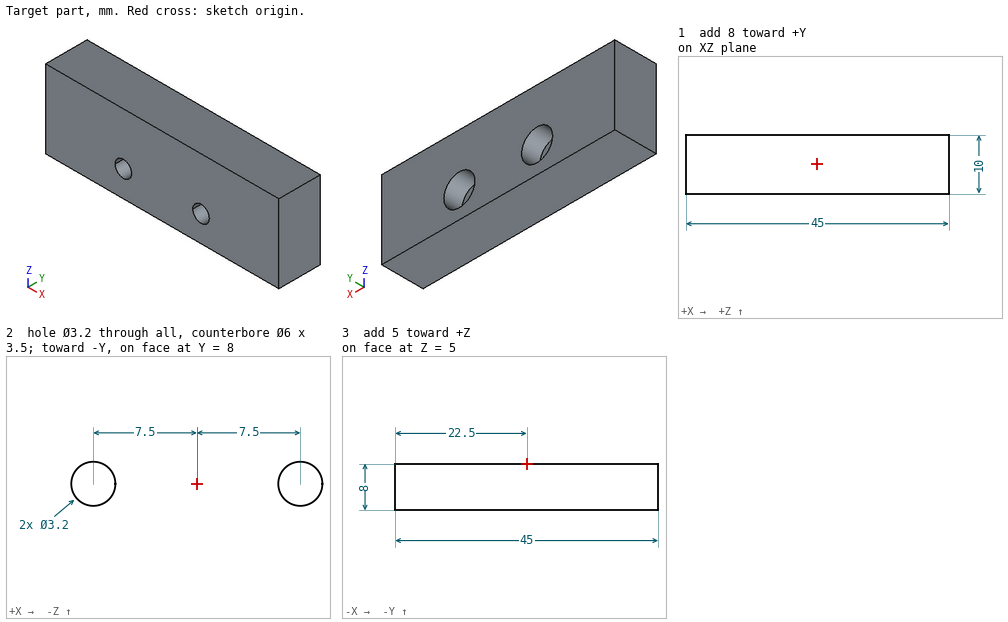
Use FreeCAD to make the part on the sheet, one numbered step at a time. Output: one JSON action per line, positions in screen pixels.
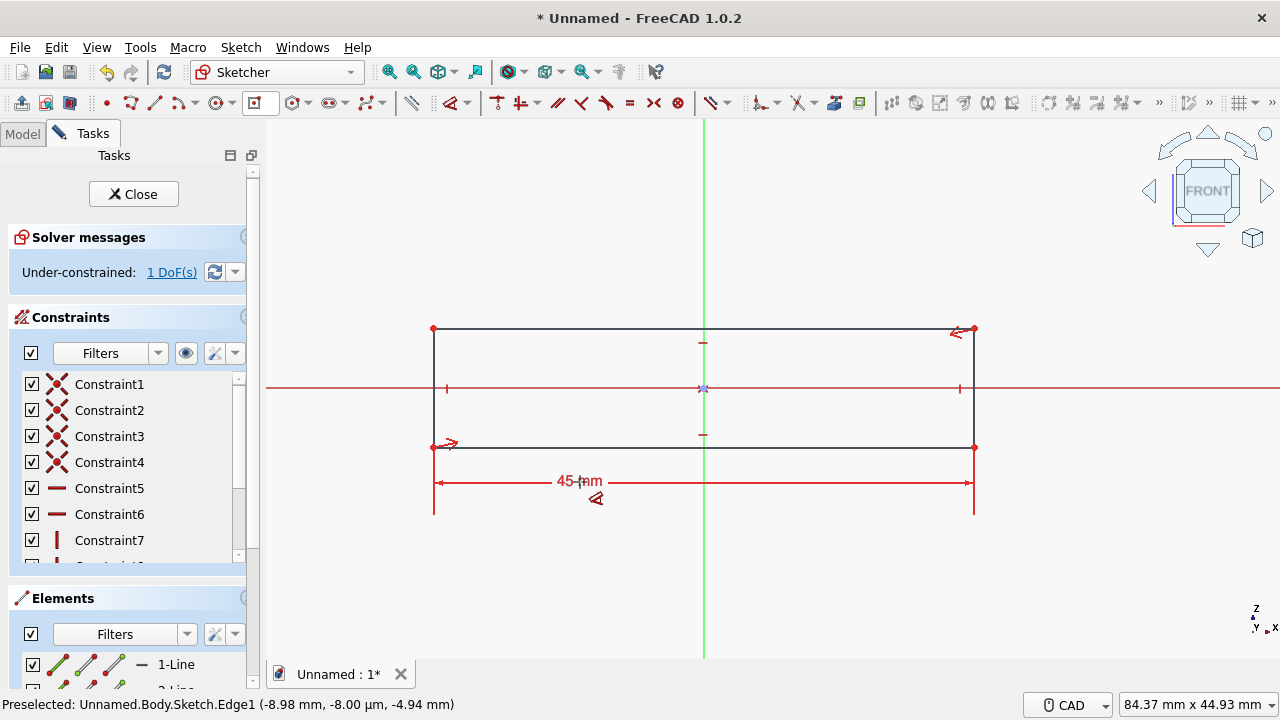
{"action": "left_click", "coordinate": [974, 412]}
{"action": "left_click", "coordinate": [1008, 361]}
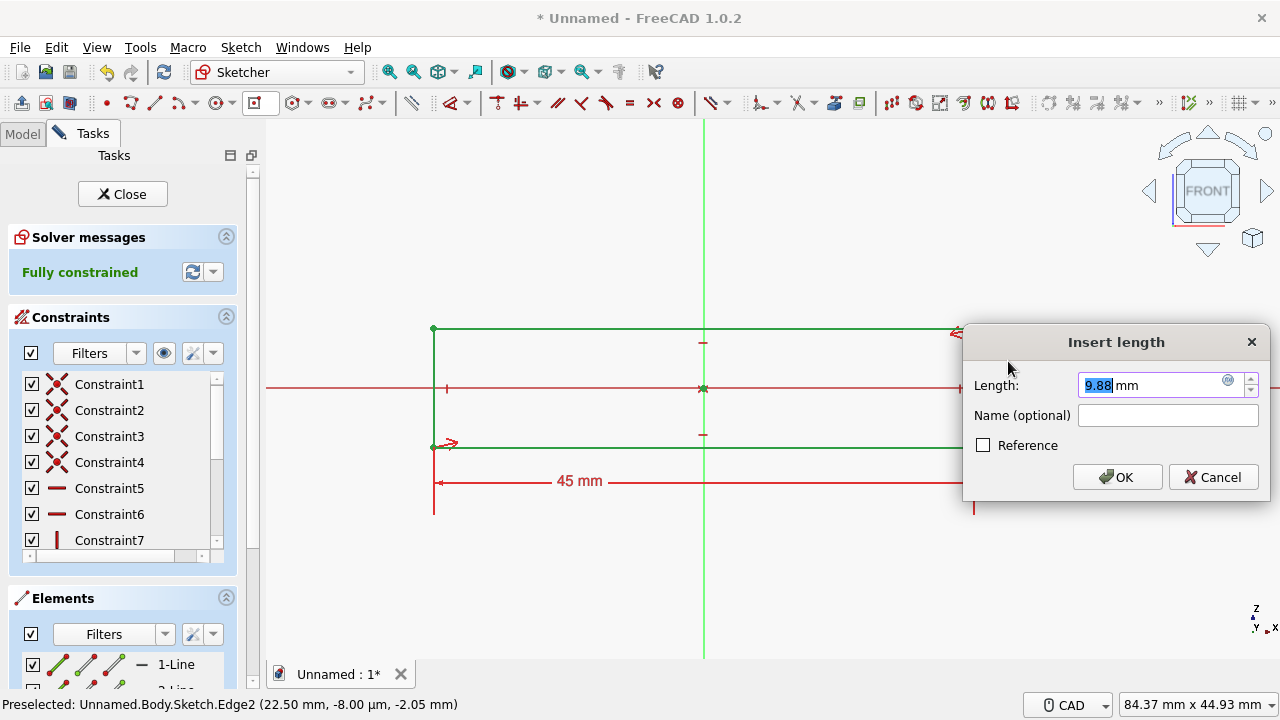
{"action": "type", "text": "10"}
{"action": "key", "text": "Return"}
{"action": "key", "text": "Escape"}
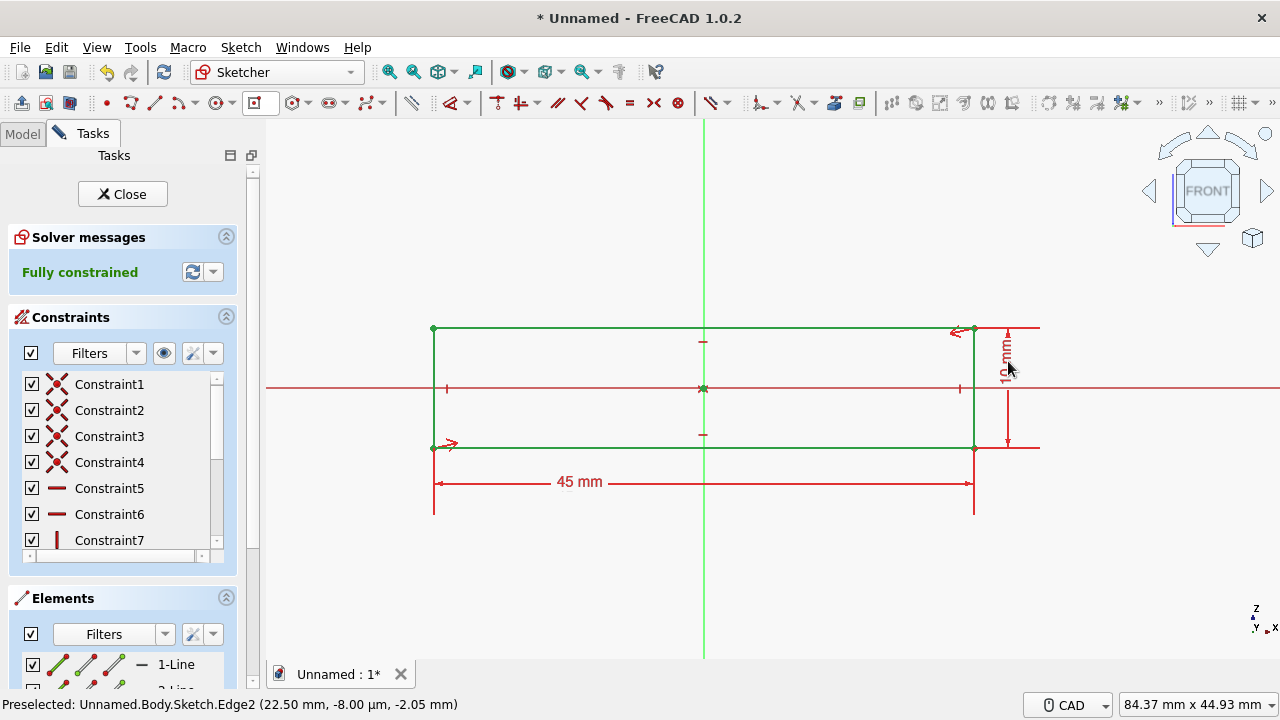
{"action": "left_click", "coordinate": [123, 194]}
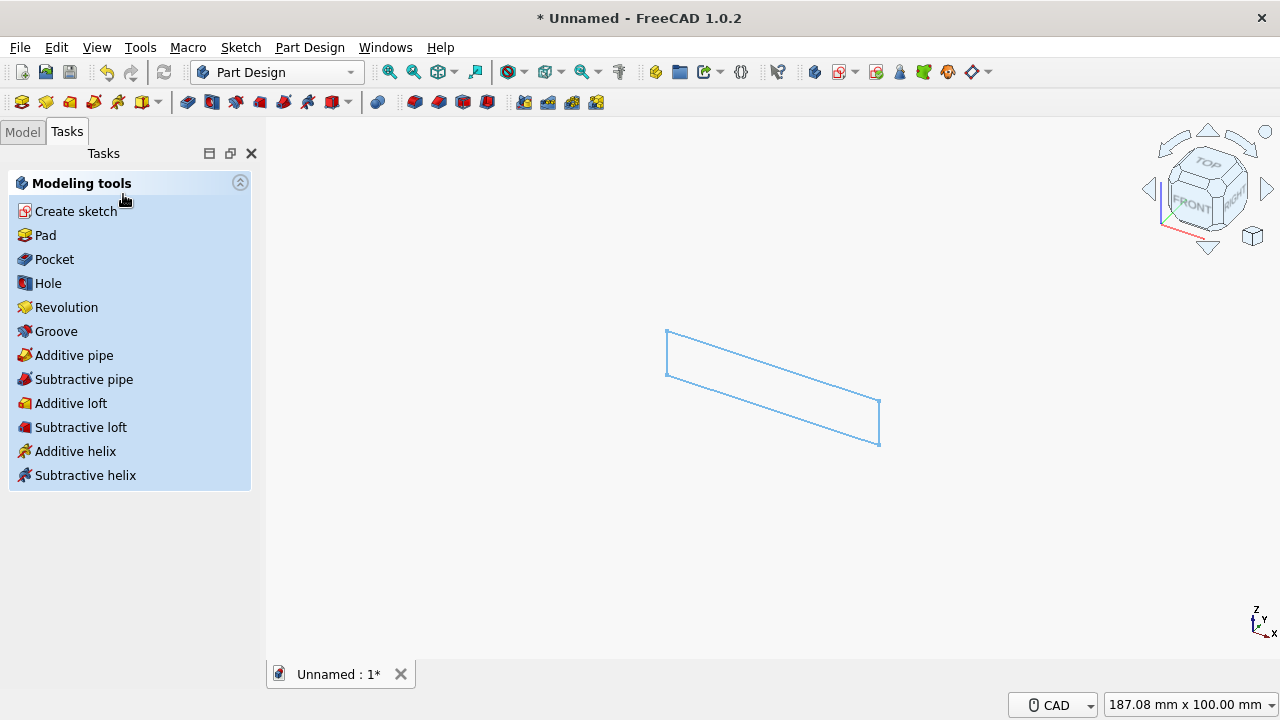
{"action": "left_click", "coordinate": [22, 102]}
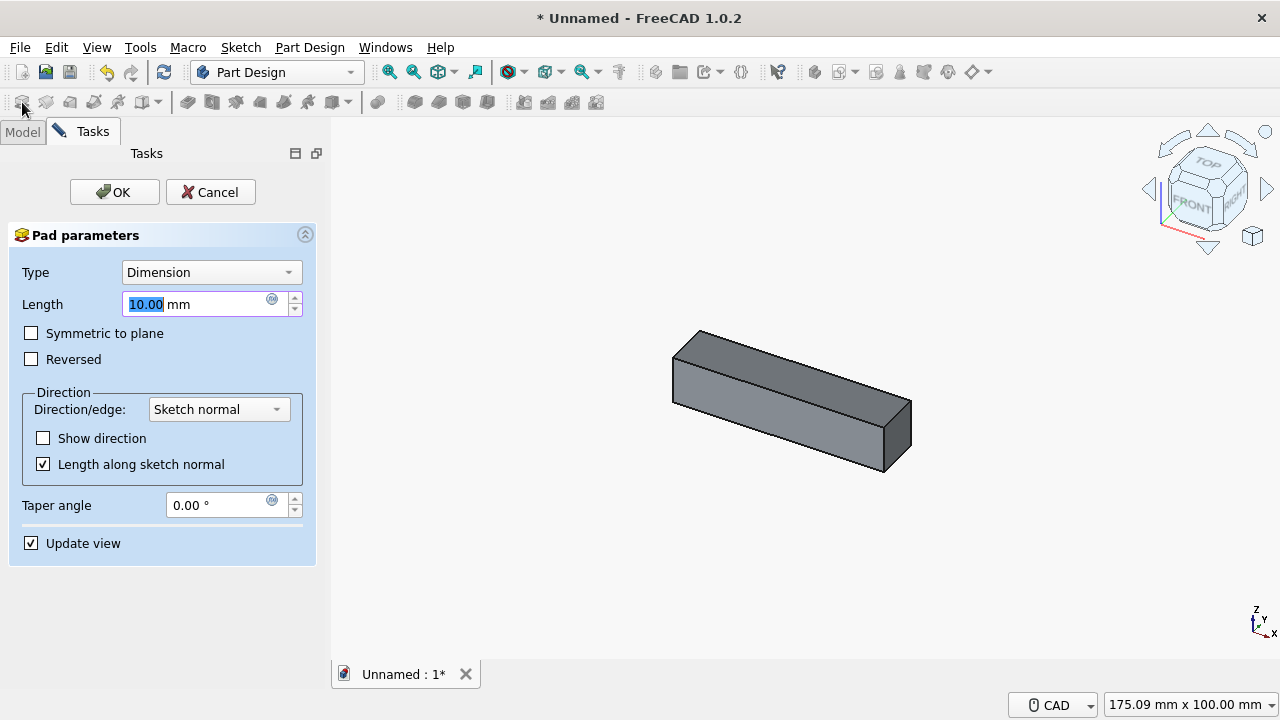
{"action": "type", "text": "8"}
{"action": "key", "text": "Tab"}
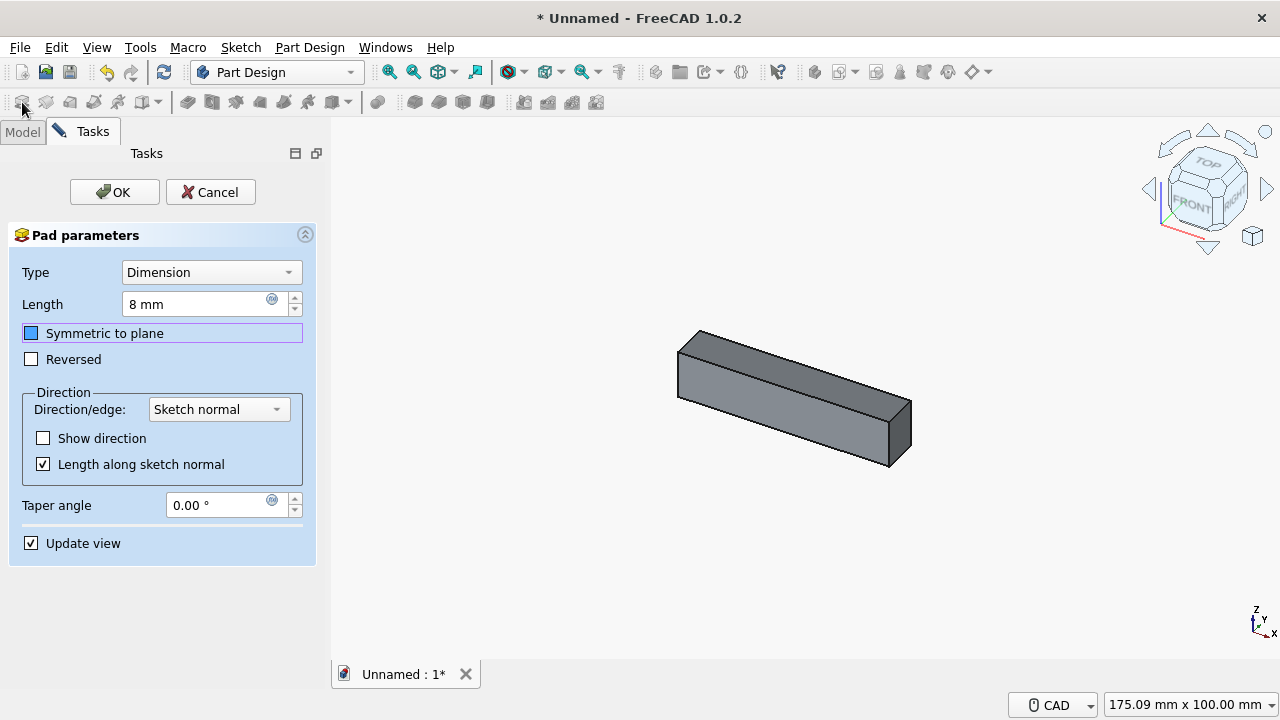
{"action": "left_click", "coordinate": [30, 359]}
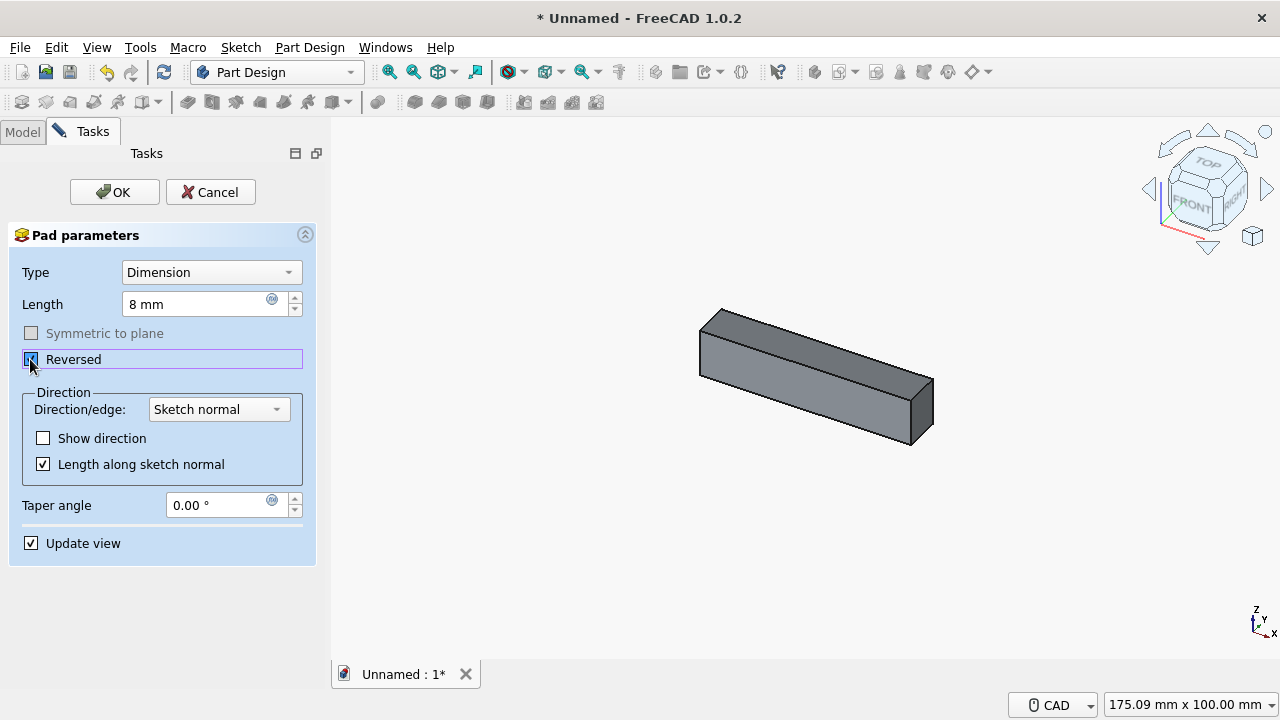
{"action": "left_click", "coordinate": [115, 192]}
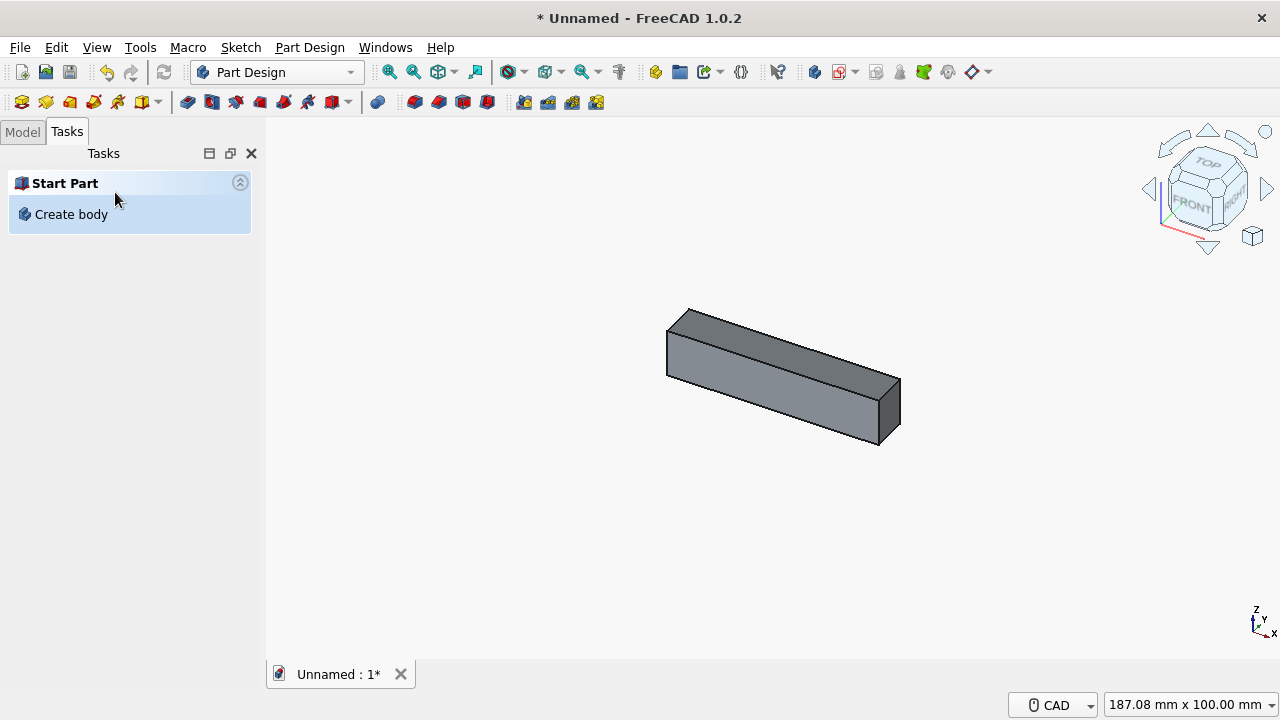
{"action": "key", "text": "v f"}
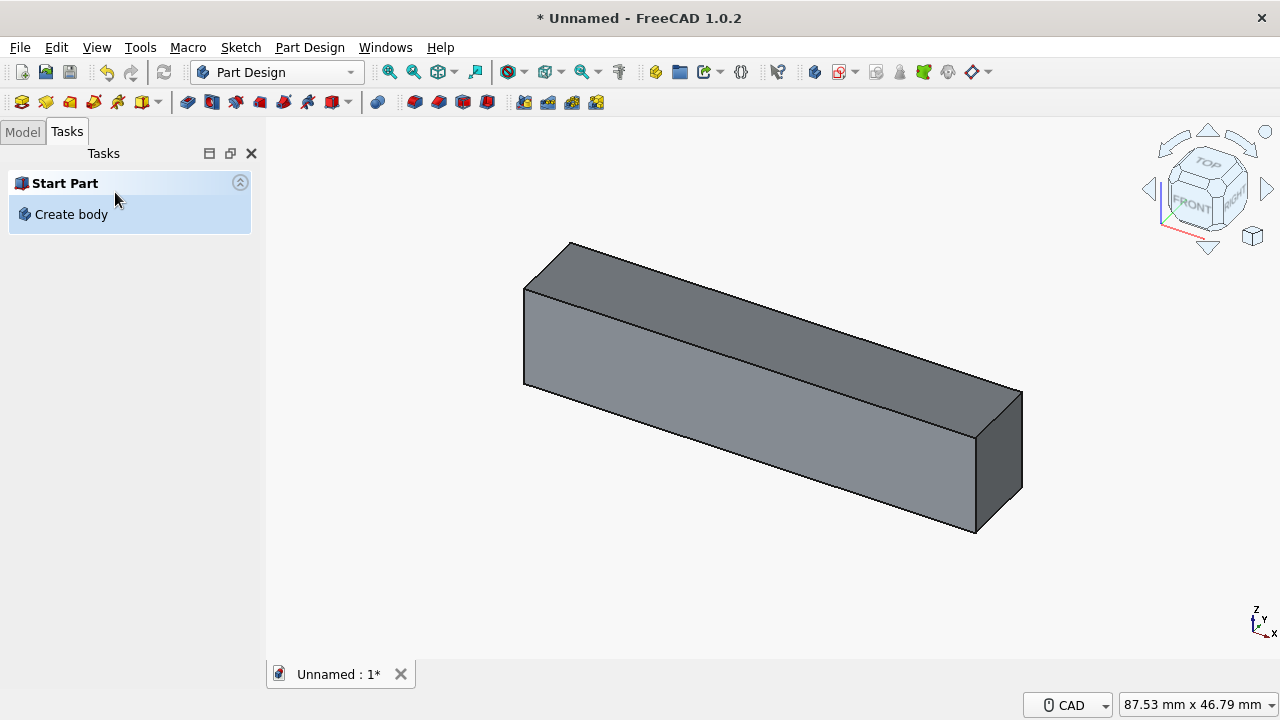
{"action": "key", "text": "4"}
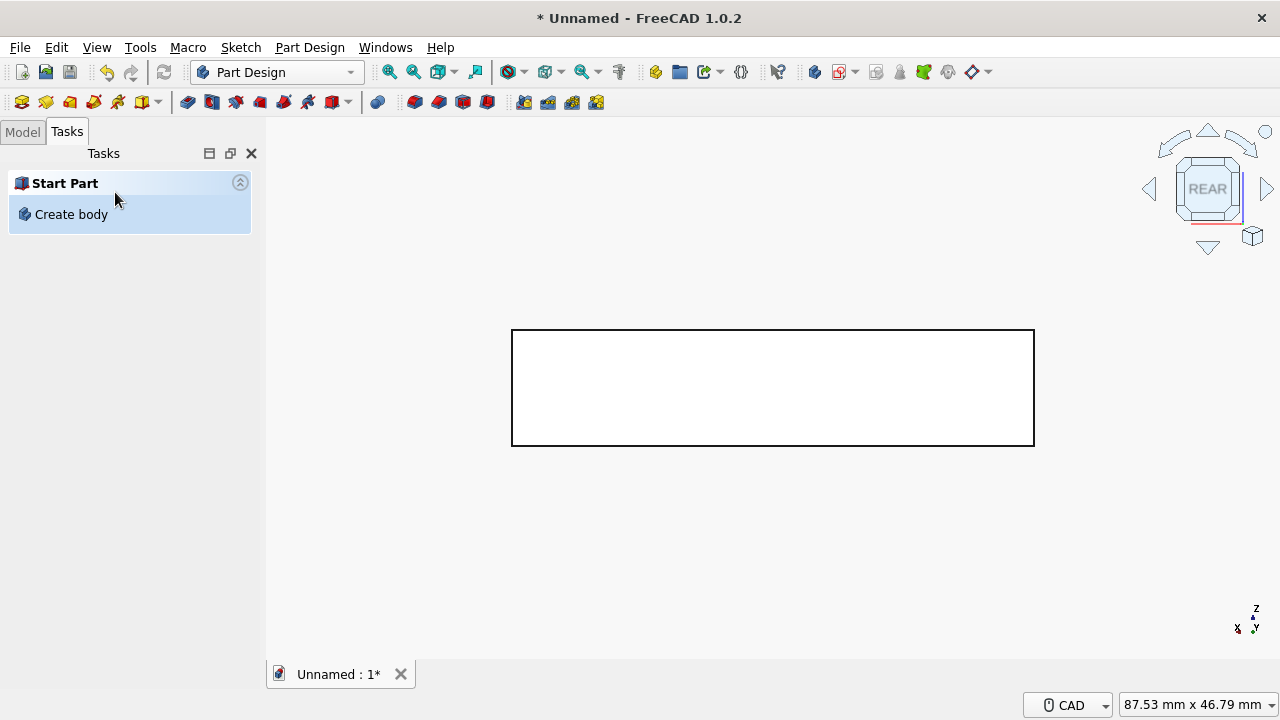
{"action": "left_click", "coordinate": [624, 387]}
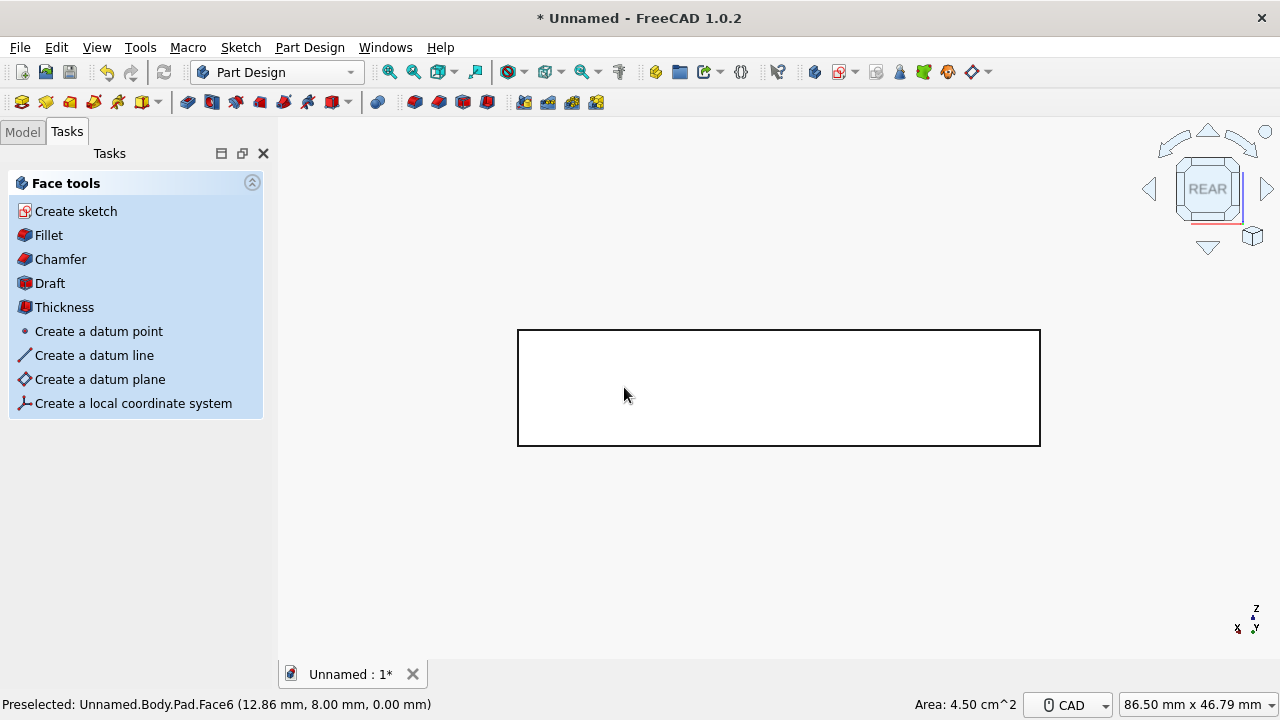
{"action": "left_click", "coordinate": [840, 72]}